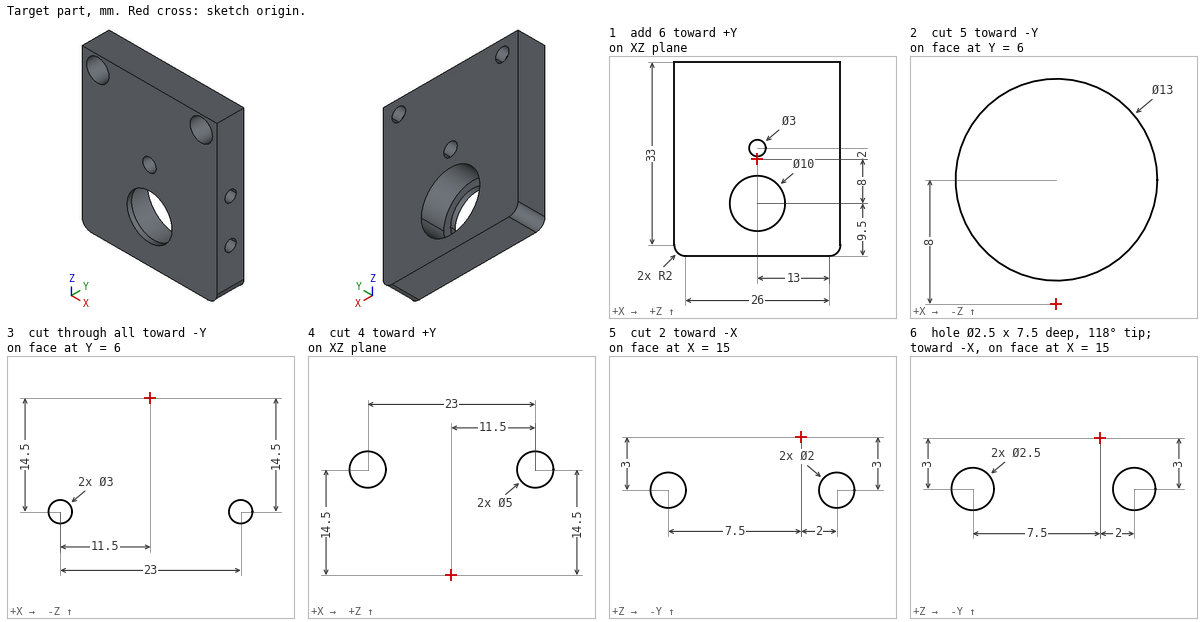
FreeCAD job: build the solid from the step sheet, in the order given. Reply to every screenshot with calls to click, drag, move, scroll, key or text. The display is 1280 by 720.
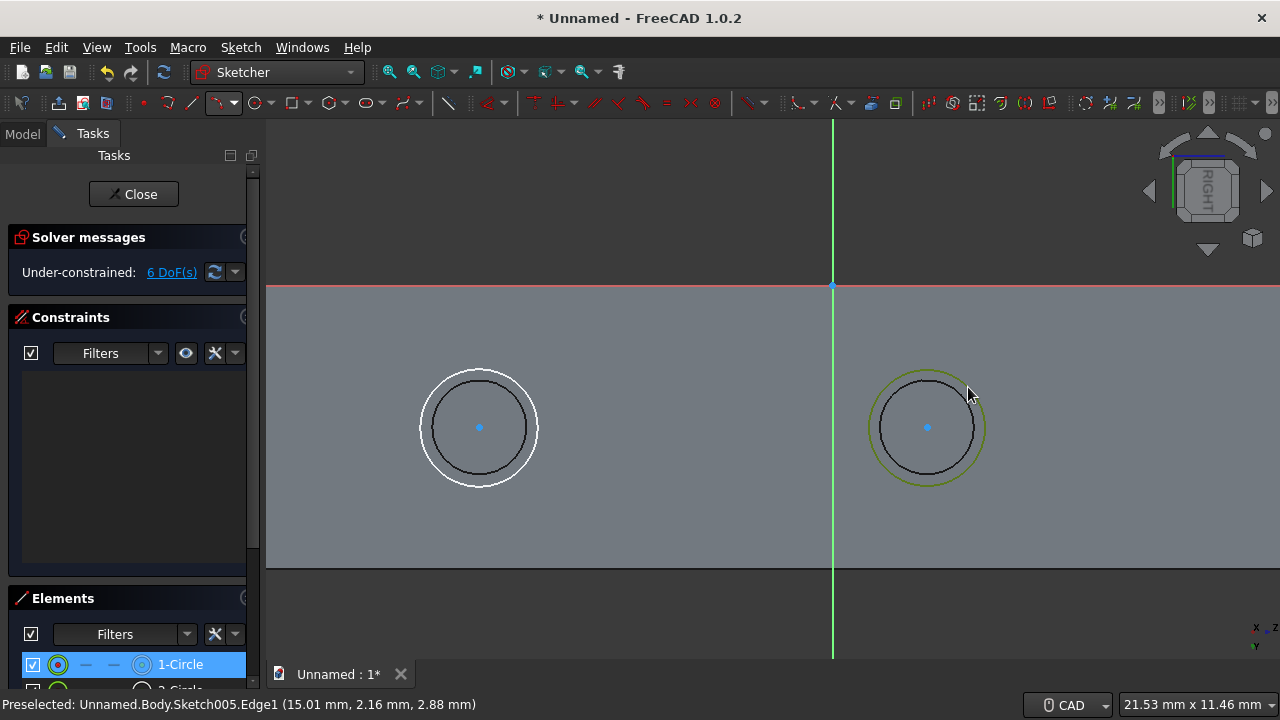
click(520, 386)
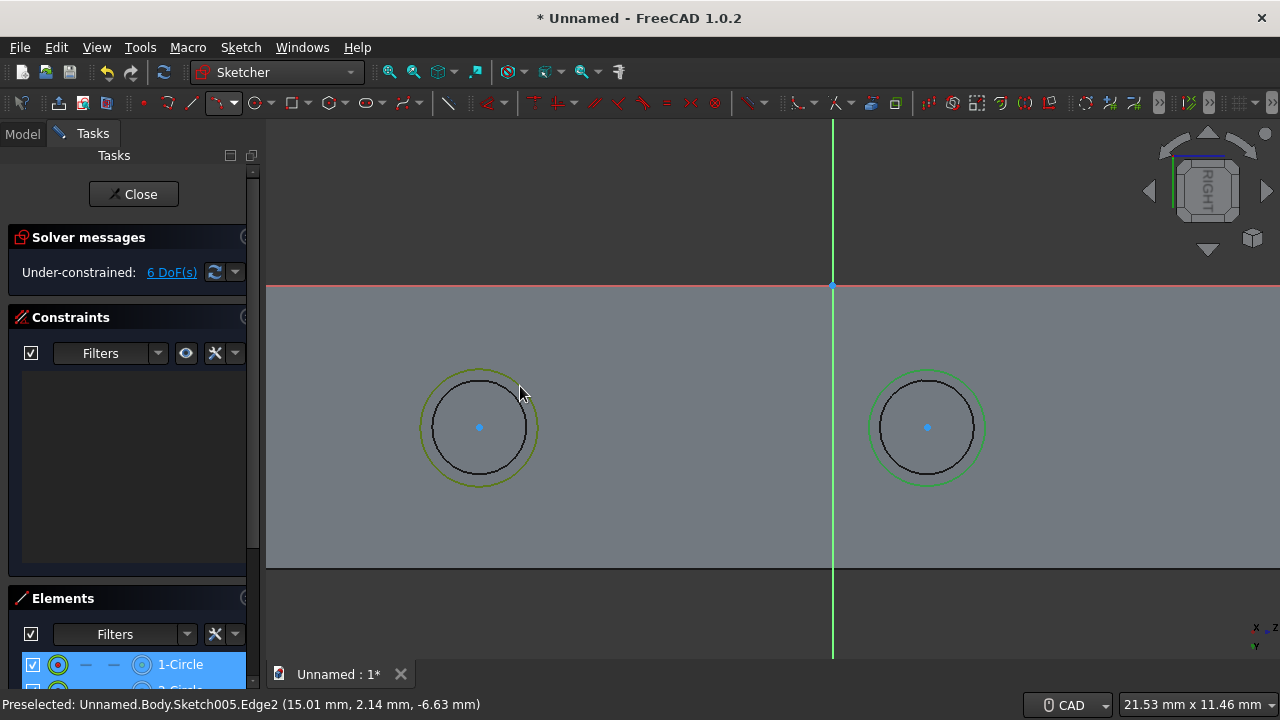
key(e)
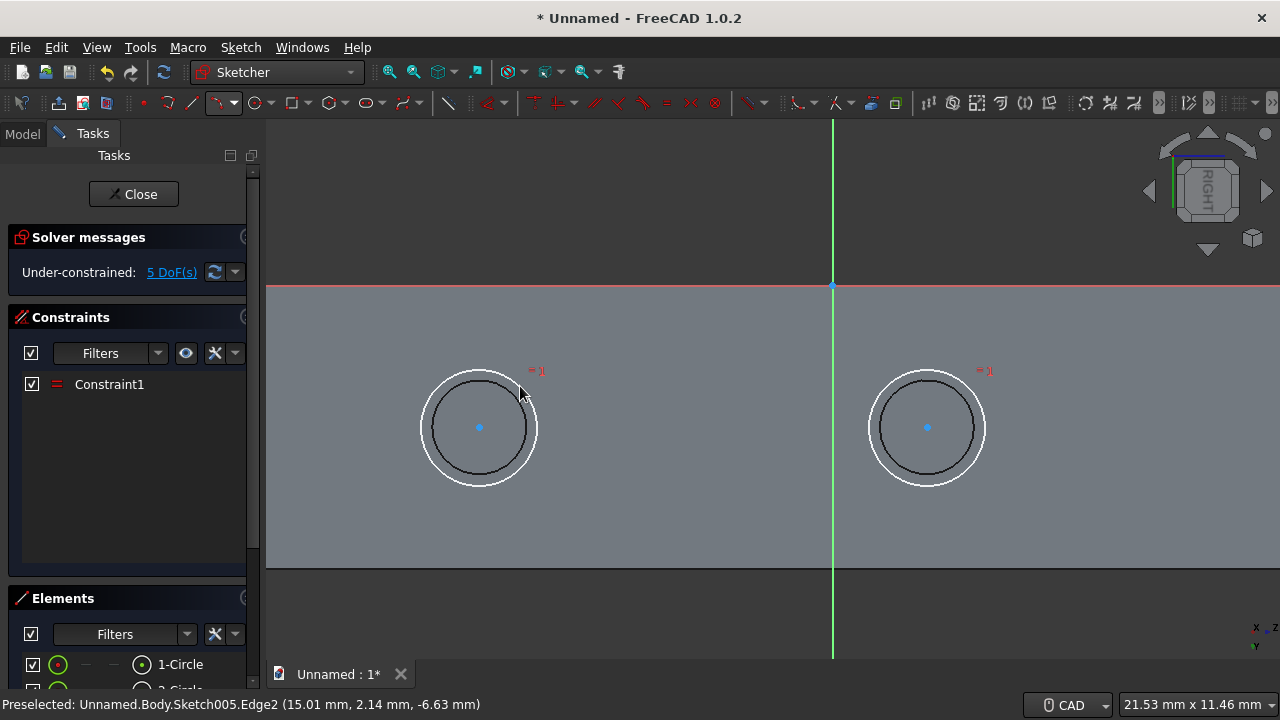
key(d)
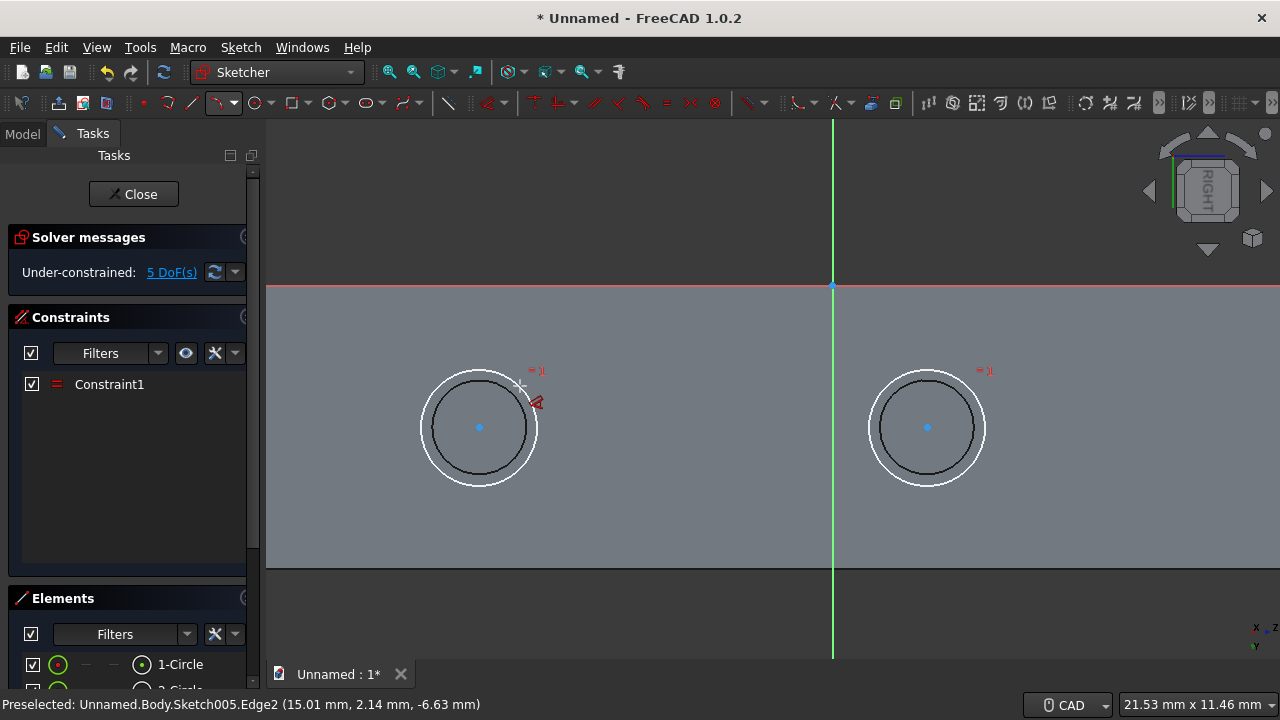
click(968, 387)
click(991, 364)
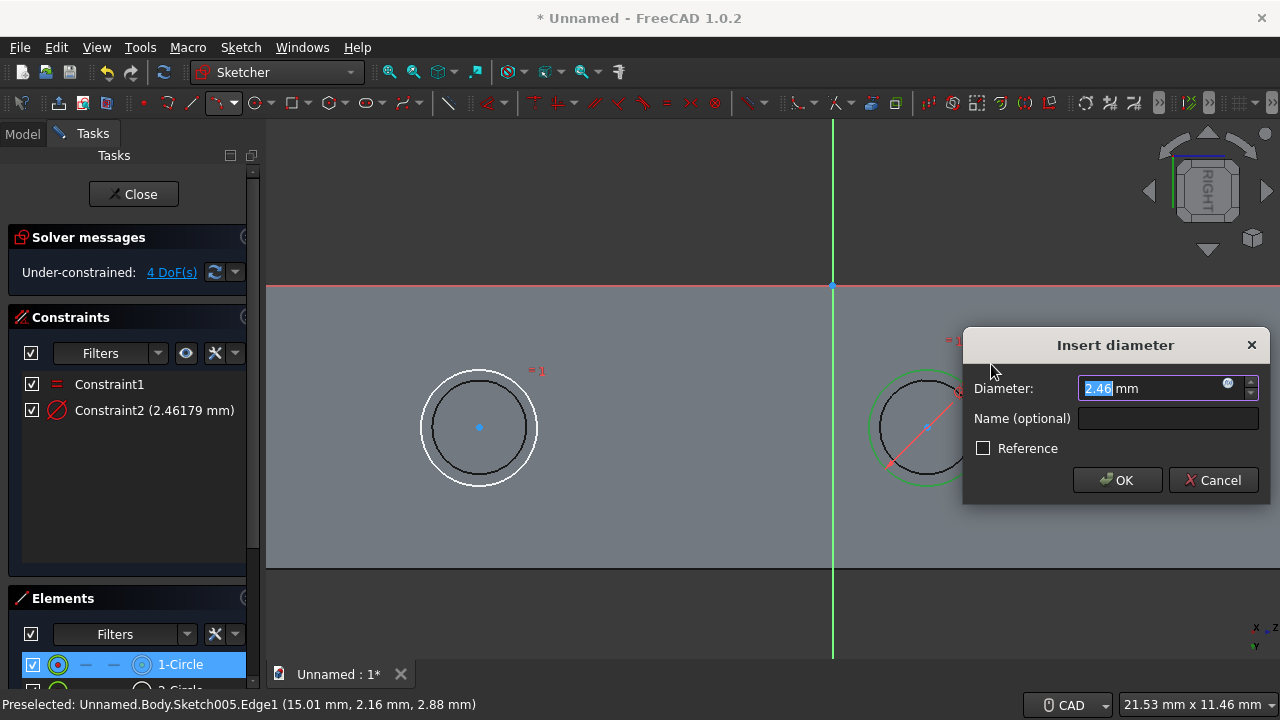
text(2.5)
key(Return)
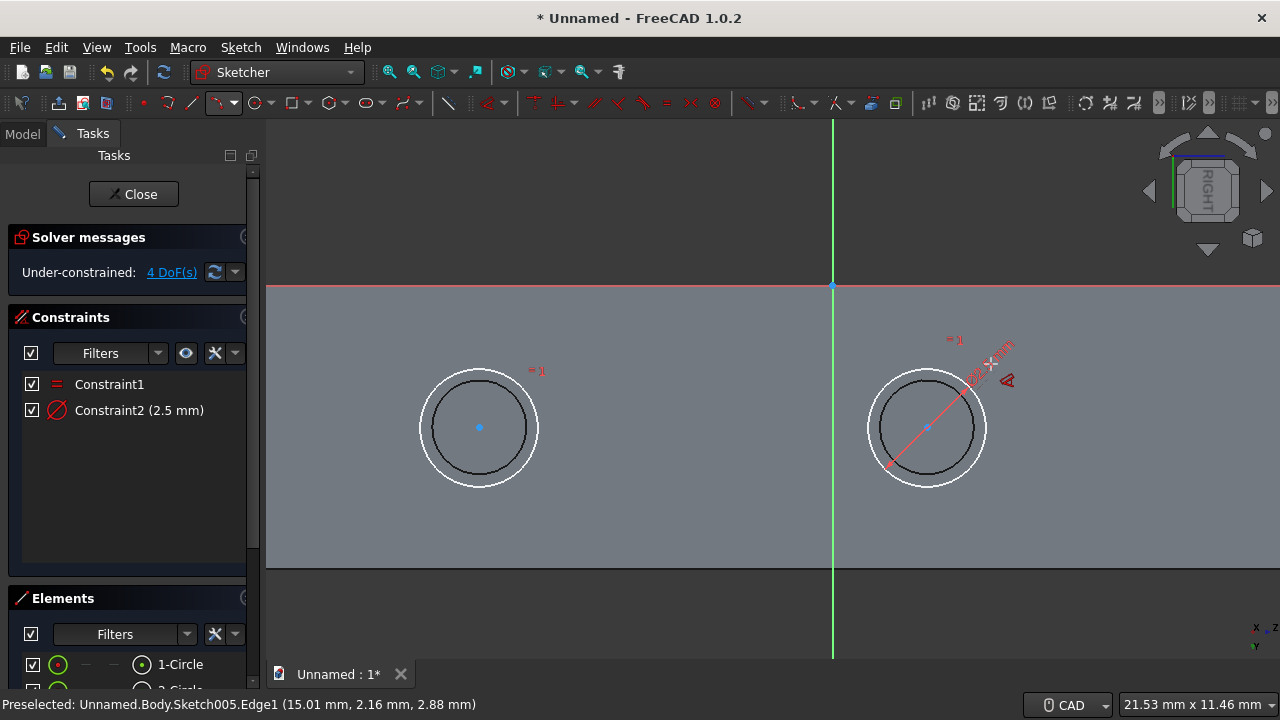
click(927, 428)
click(880, 252)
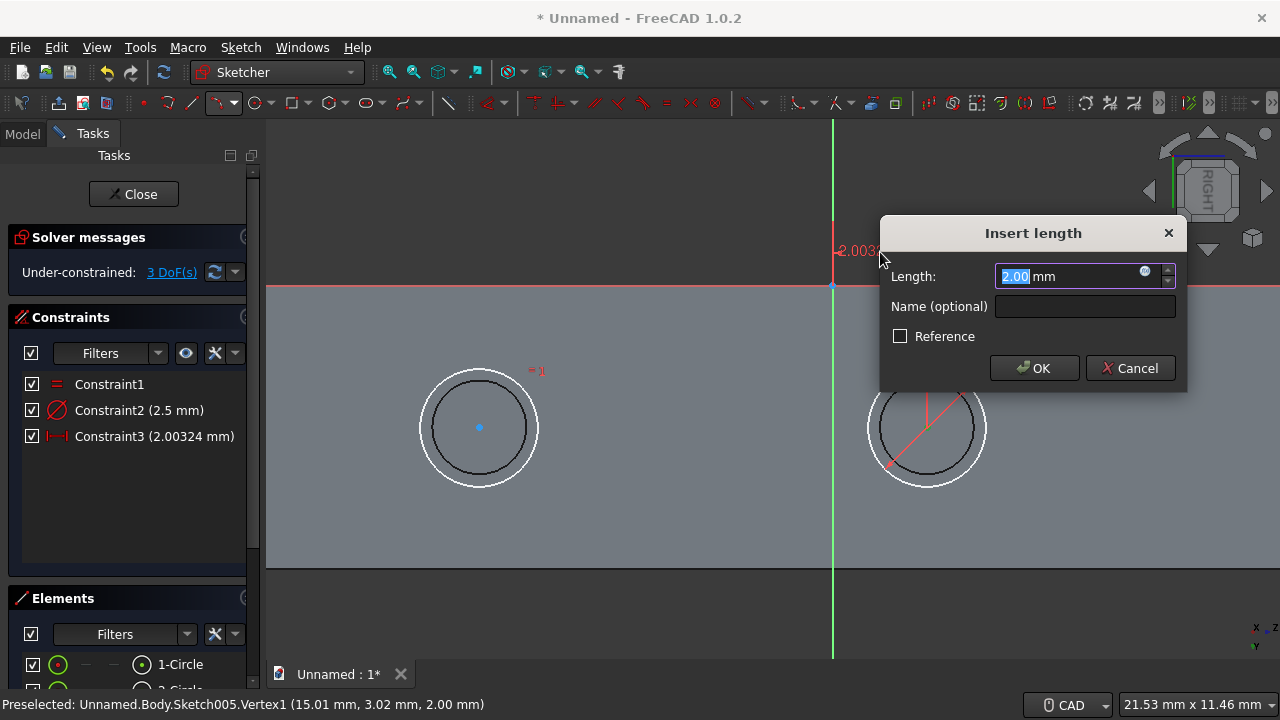
text(2)
key(Return)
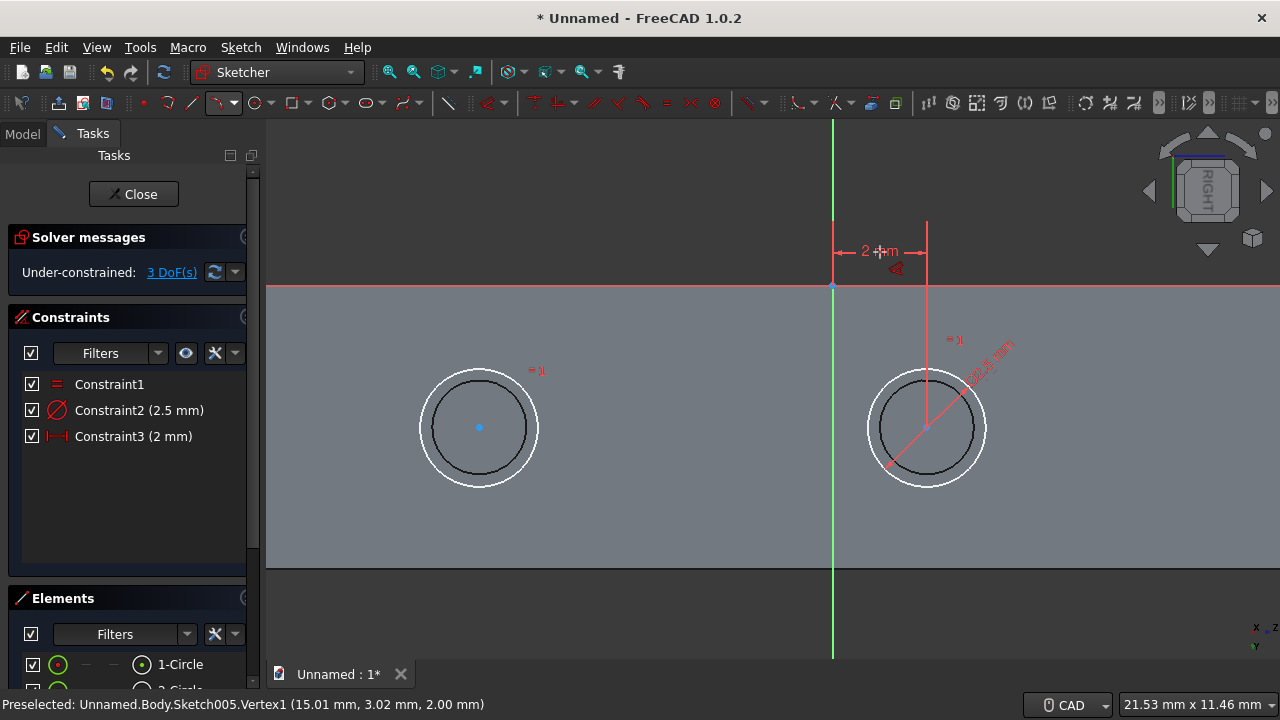
click(927, 428)
click(961, 324)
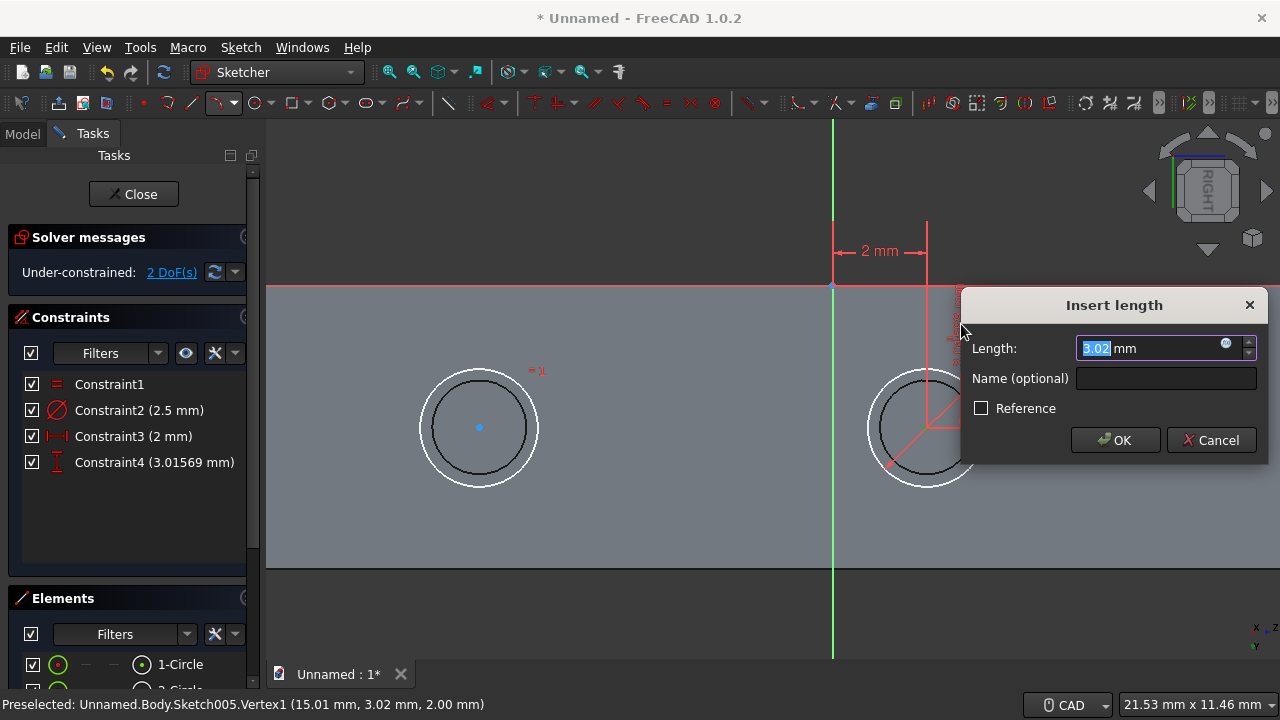
text(3)
key(Return)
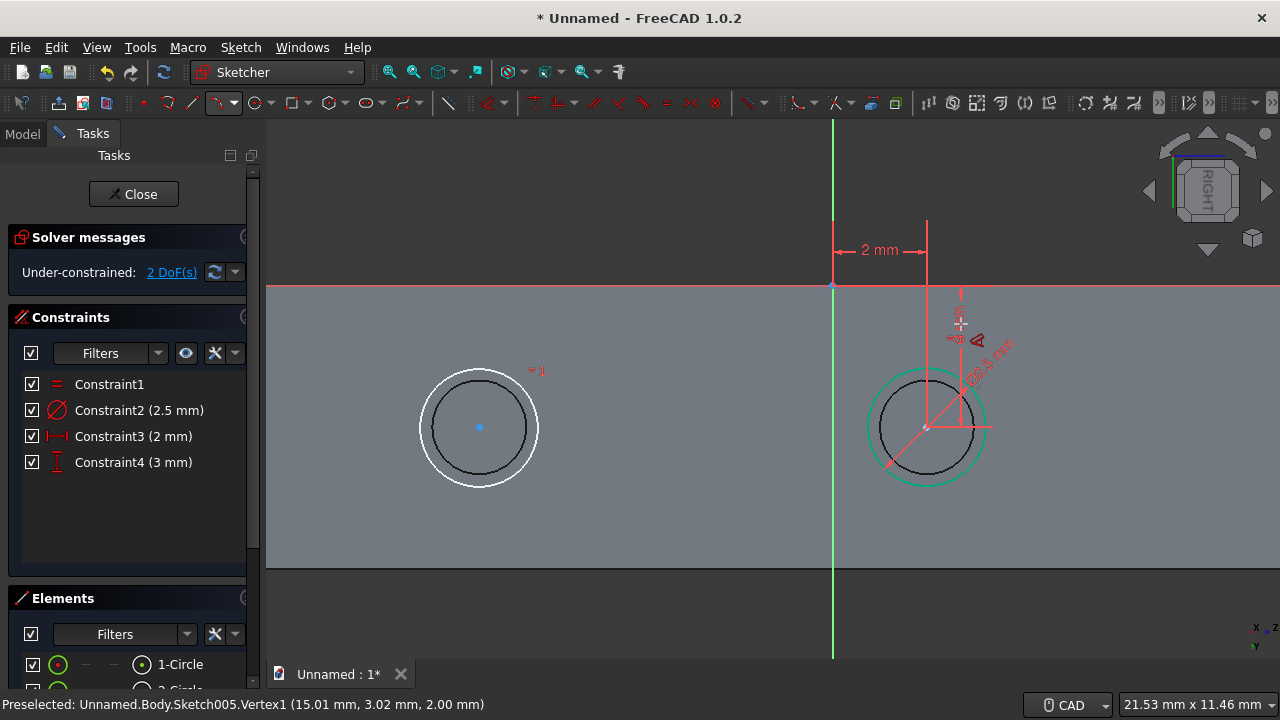
click(479, 428)
click(445, 357)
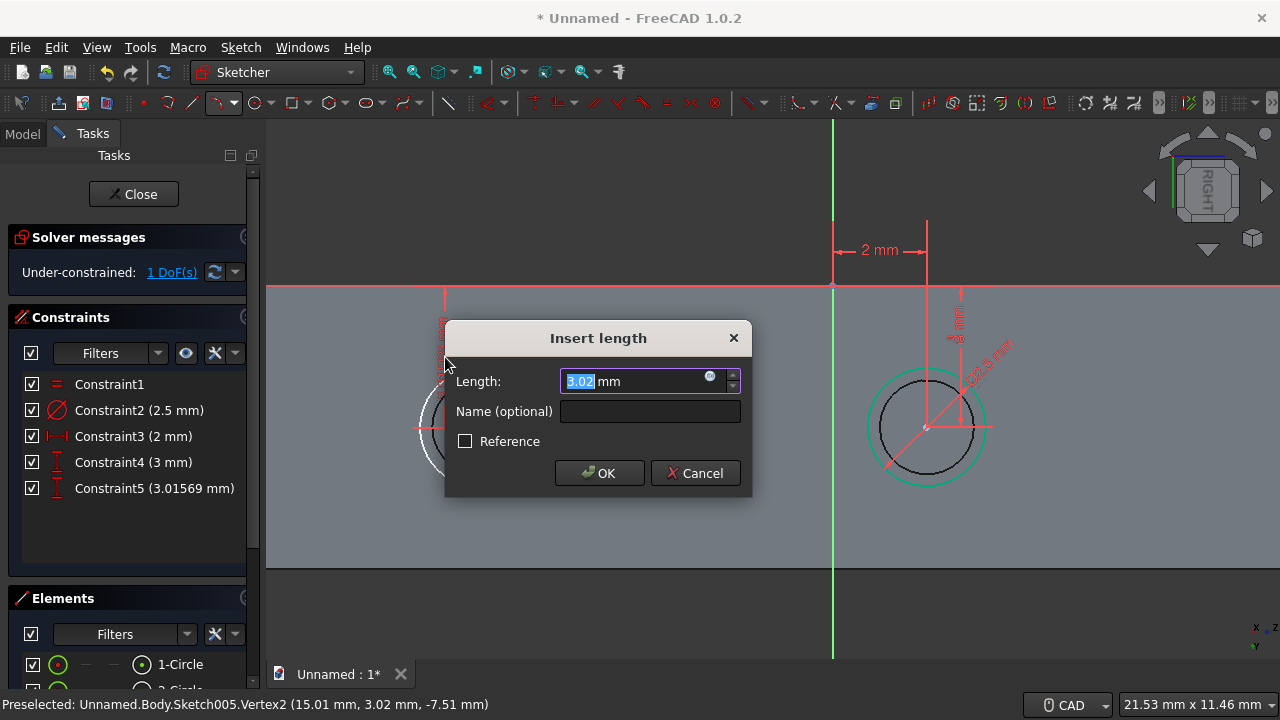
text(3)
key(Return)